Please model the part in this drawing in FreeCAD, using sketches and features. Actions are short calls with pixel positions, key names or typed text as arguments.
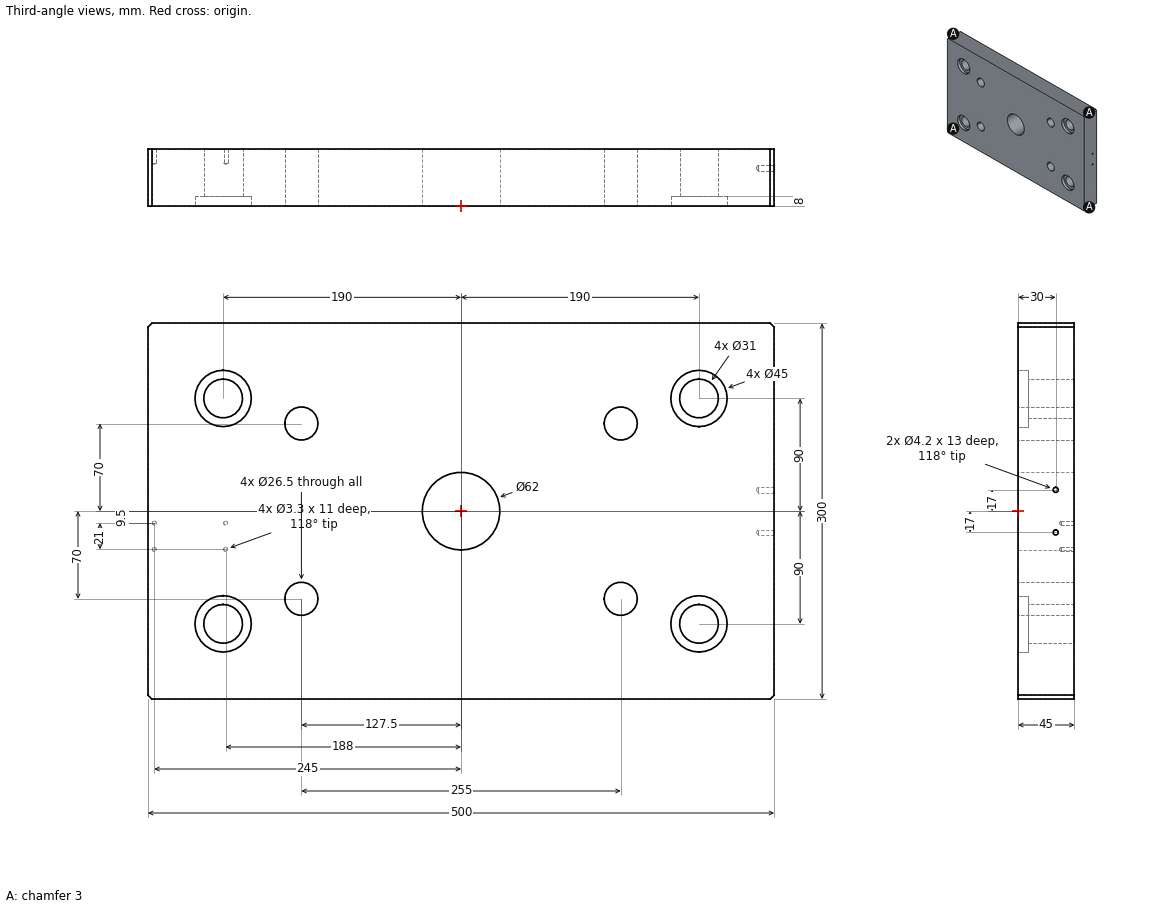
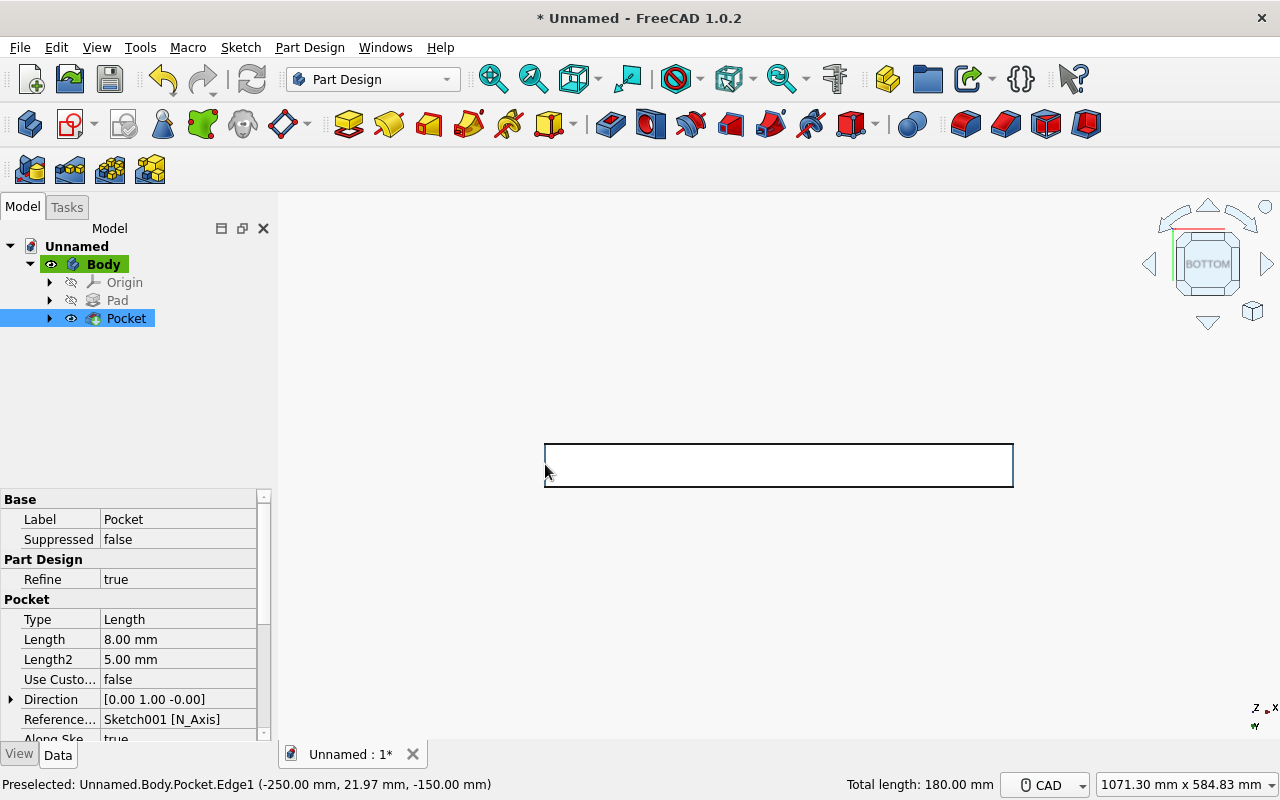
click(1006, 124)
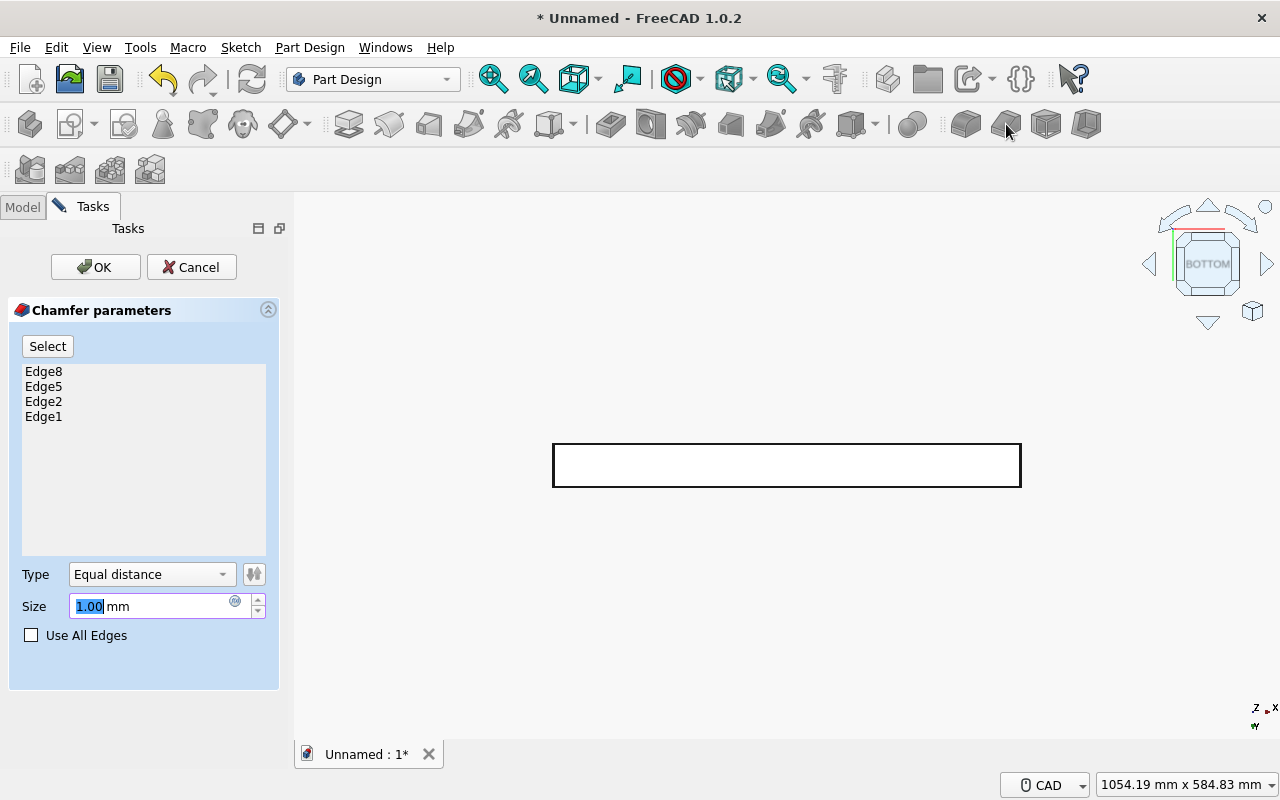
text(3)
key(Tab)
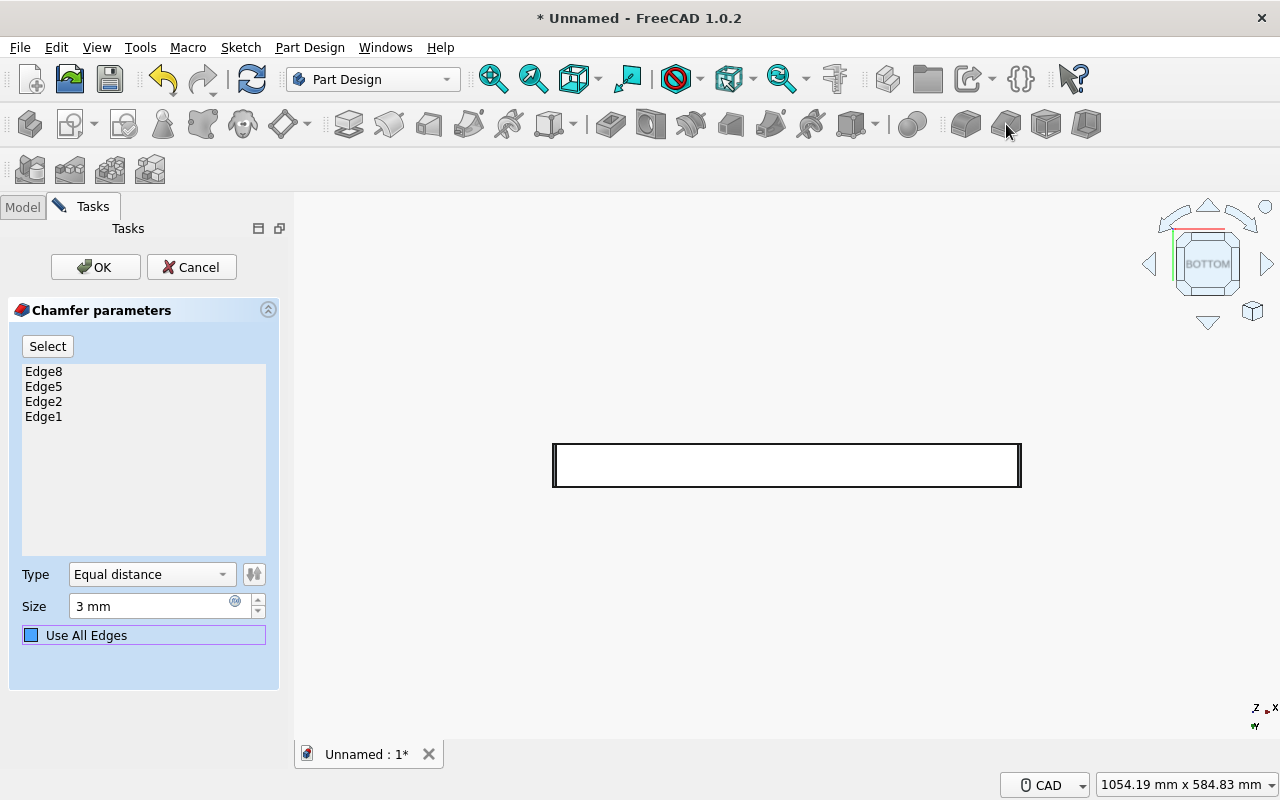
click(96, 267)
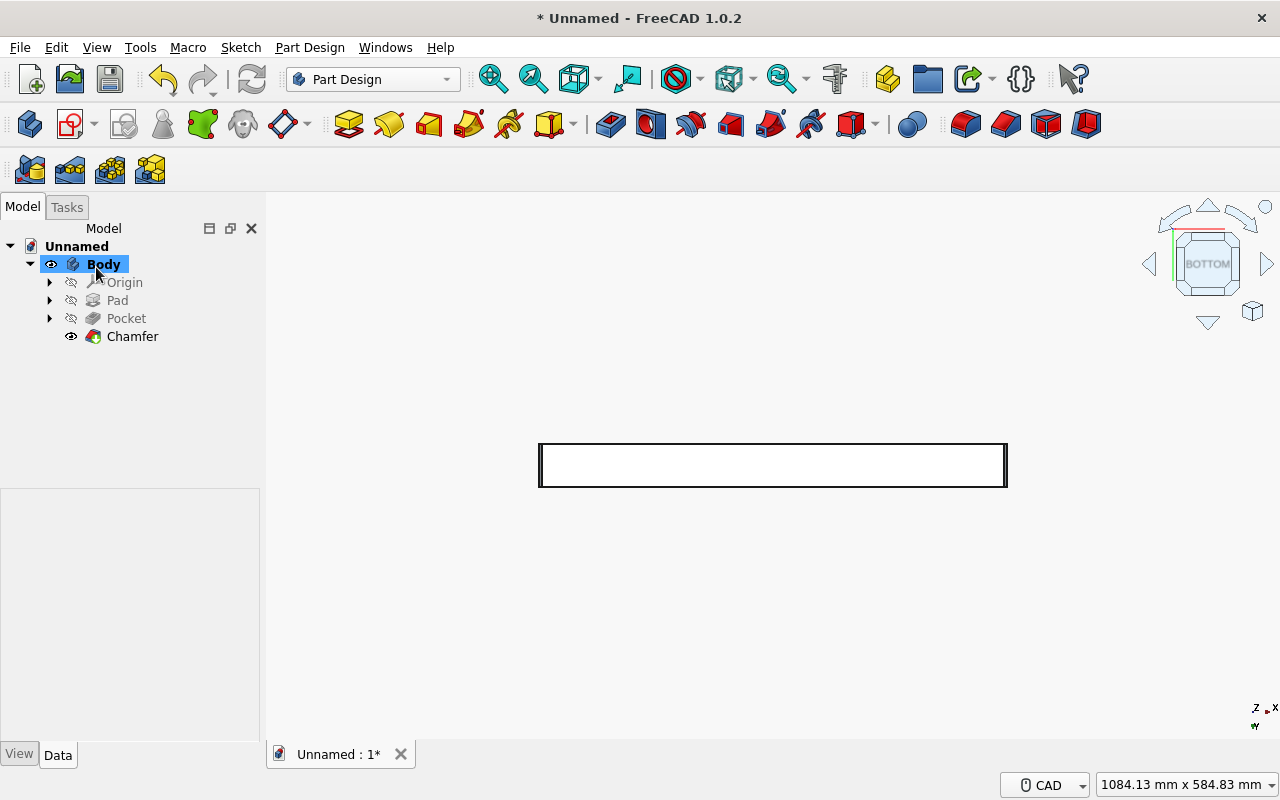
key(4)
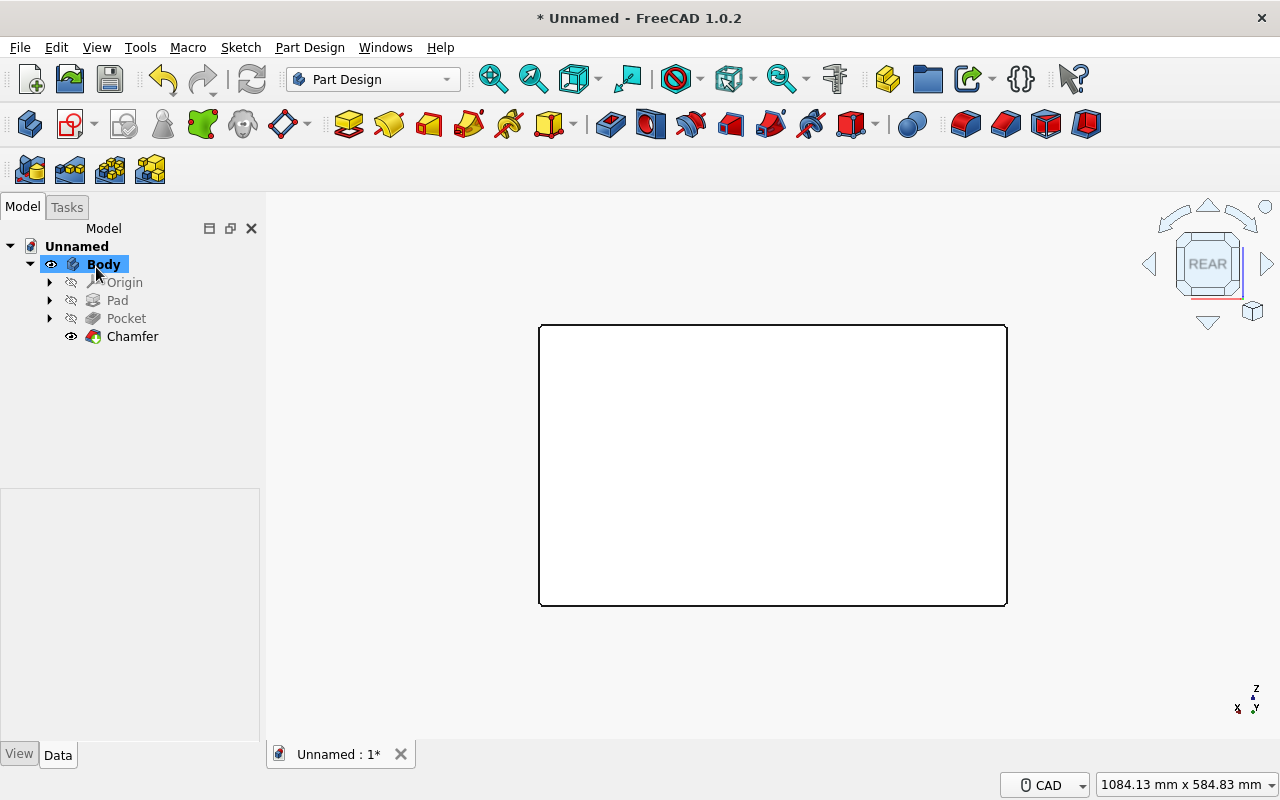
click(706, 465)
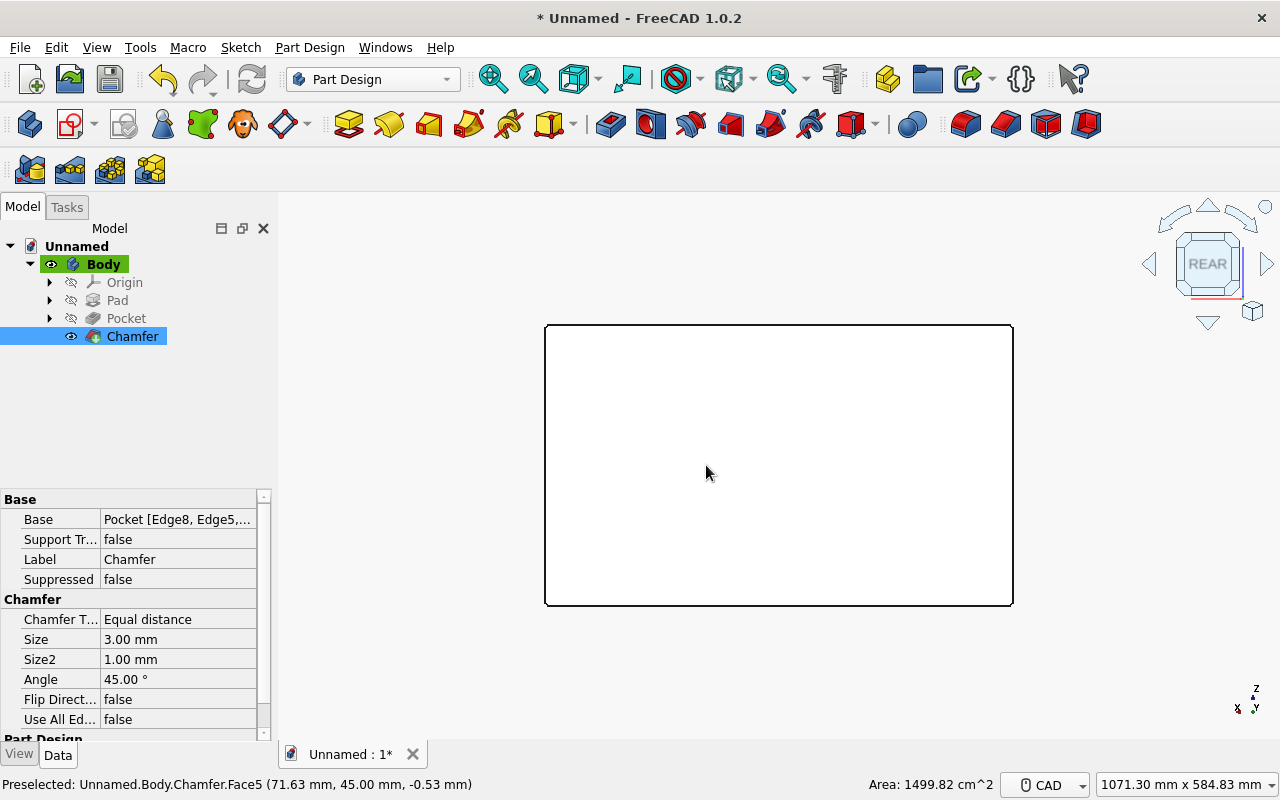
click(70, 124)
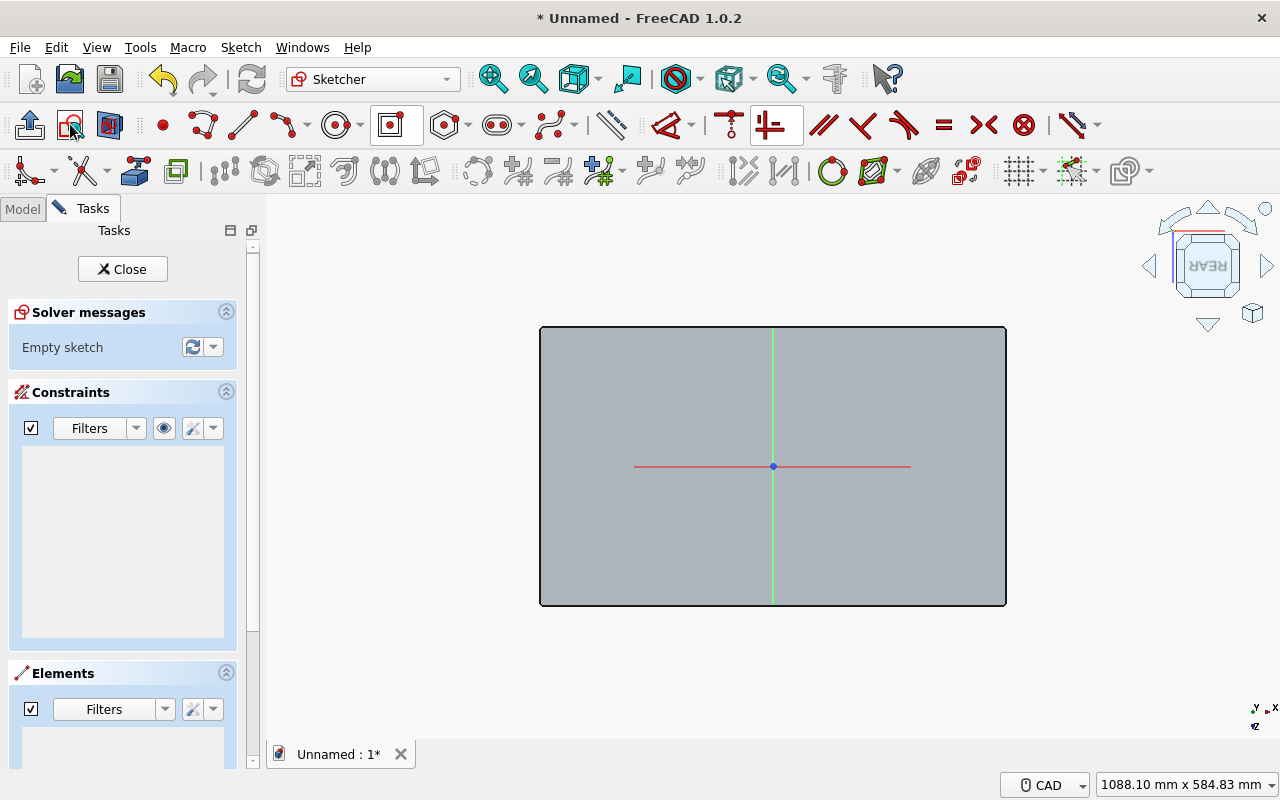
scroll(912, 466, up, 2)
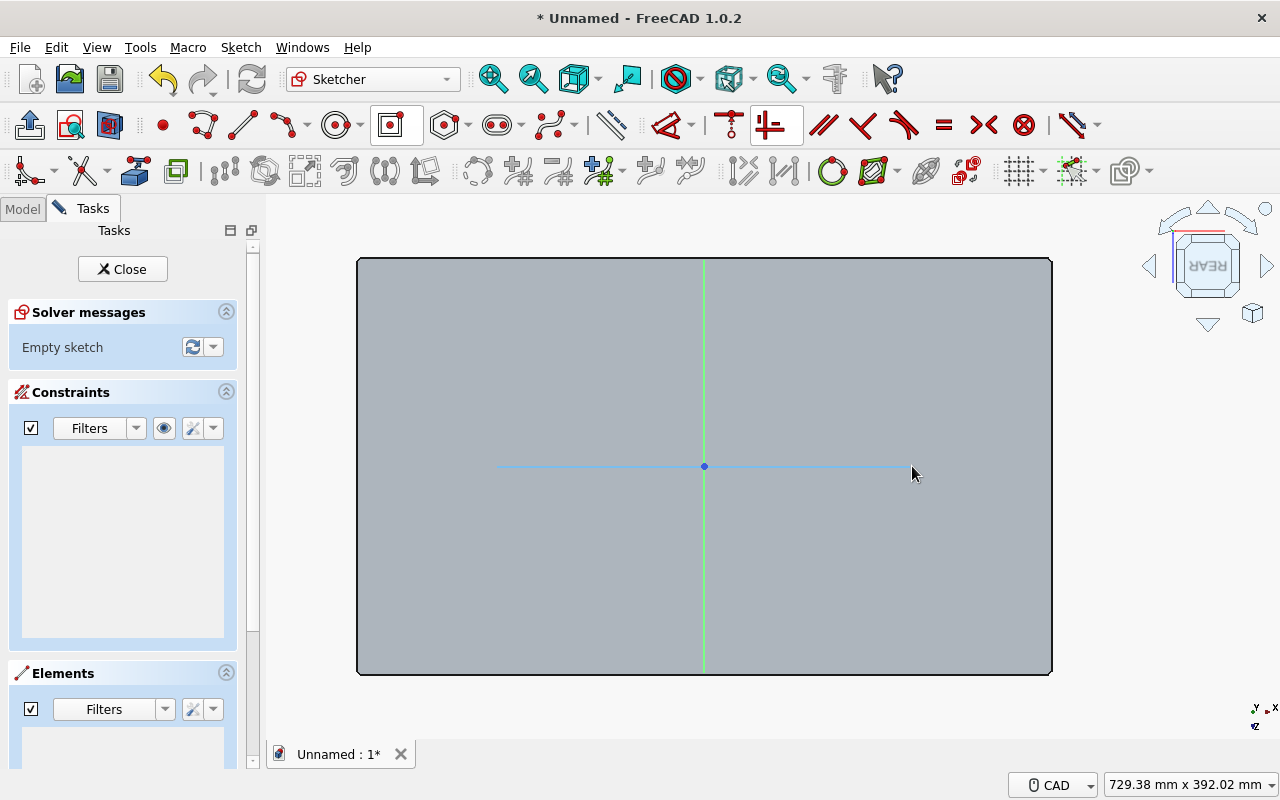
key(g)
key(c)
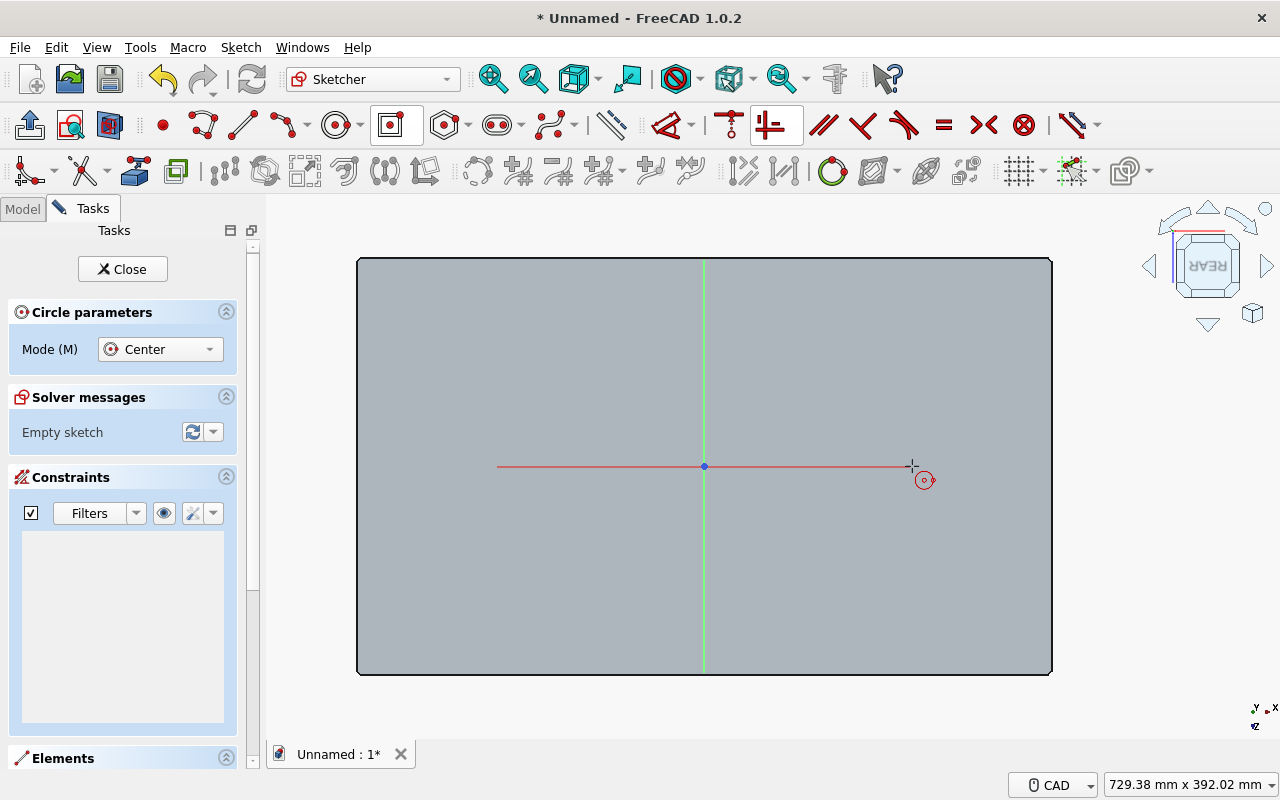
click(968, 592)
click(984, 576)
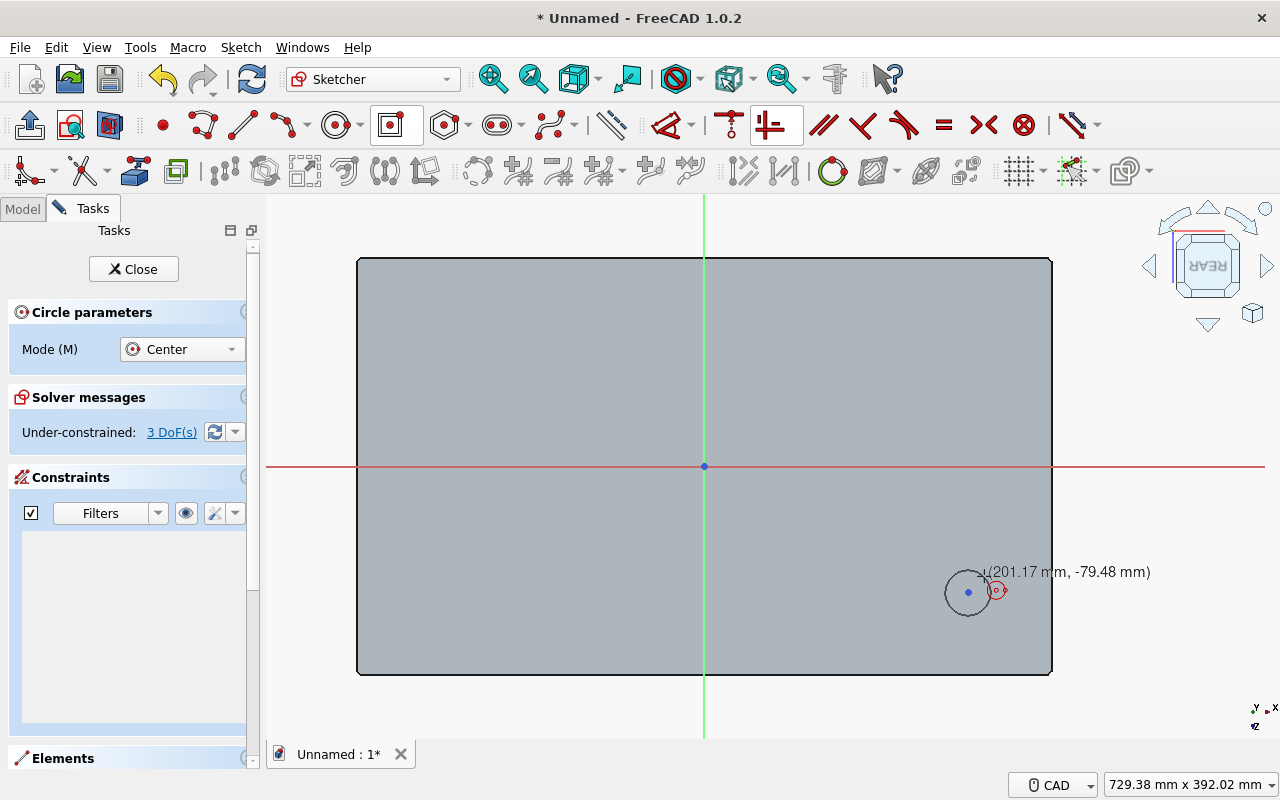
click(968, 341)
click(984, 326)